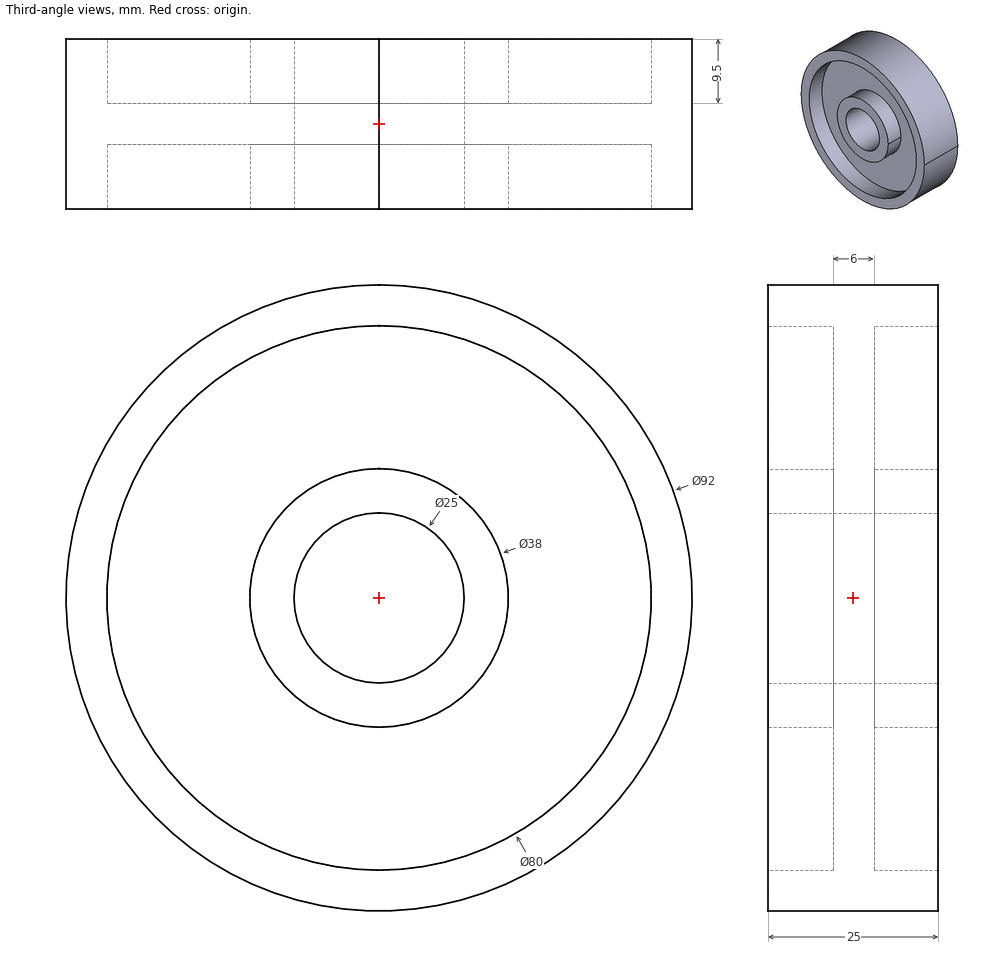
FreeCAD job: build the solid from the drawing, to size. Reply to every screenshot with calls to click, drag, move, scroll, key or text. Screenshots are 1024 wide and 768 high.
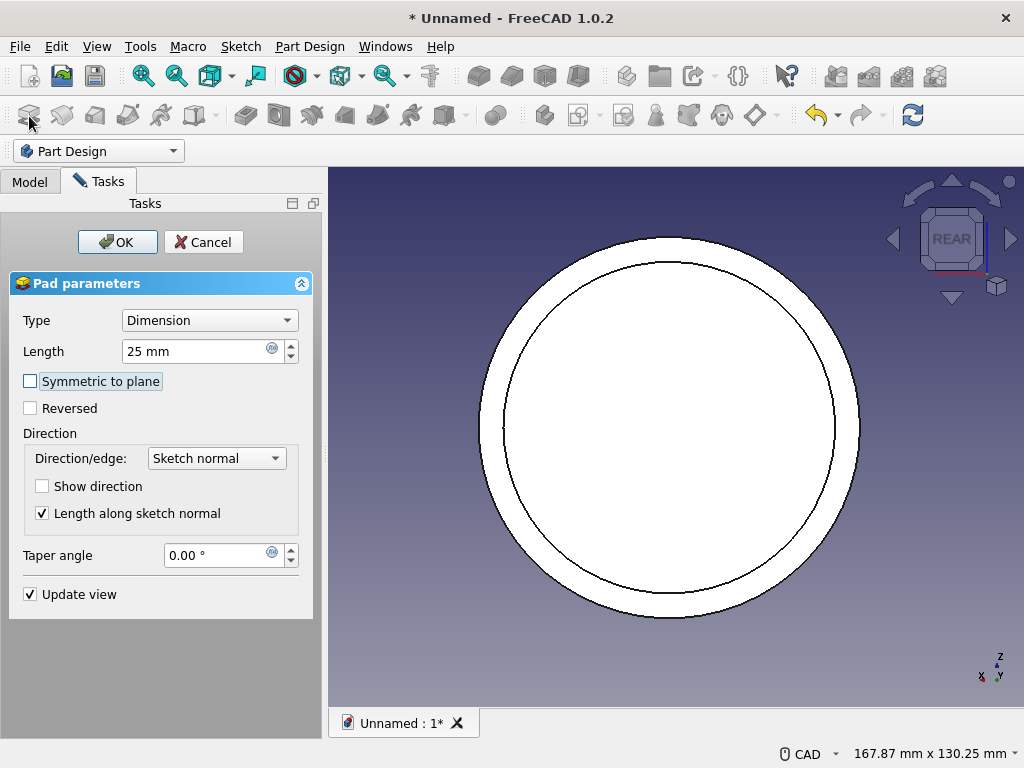
click(31, 408)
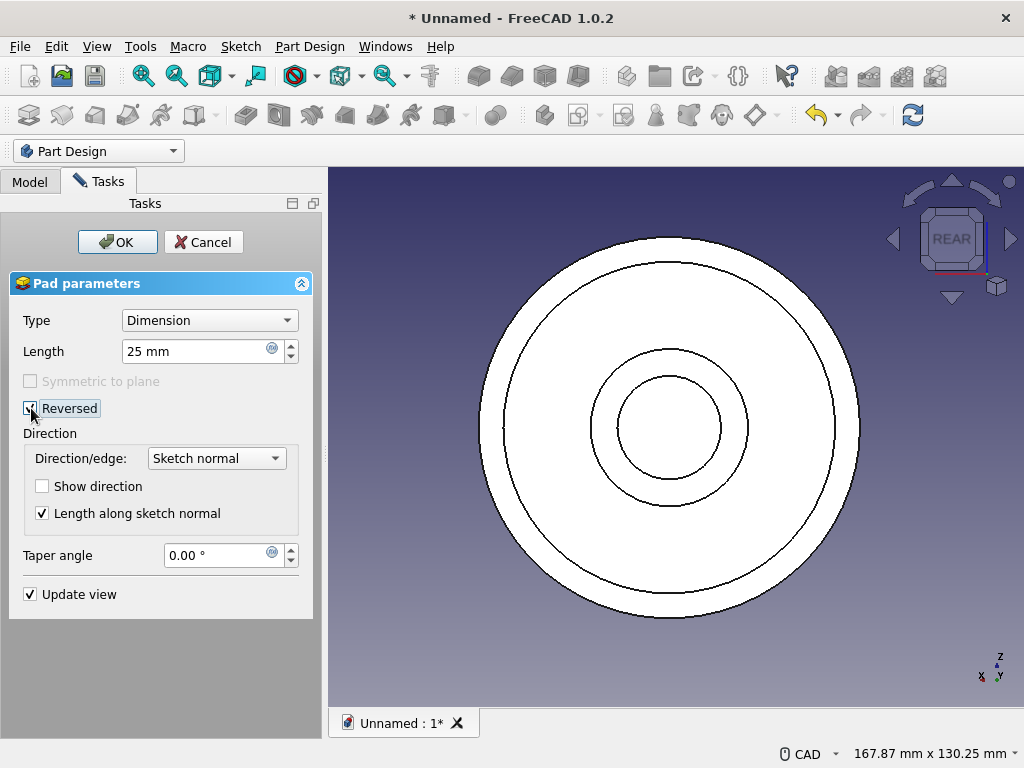
click(118, 242)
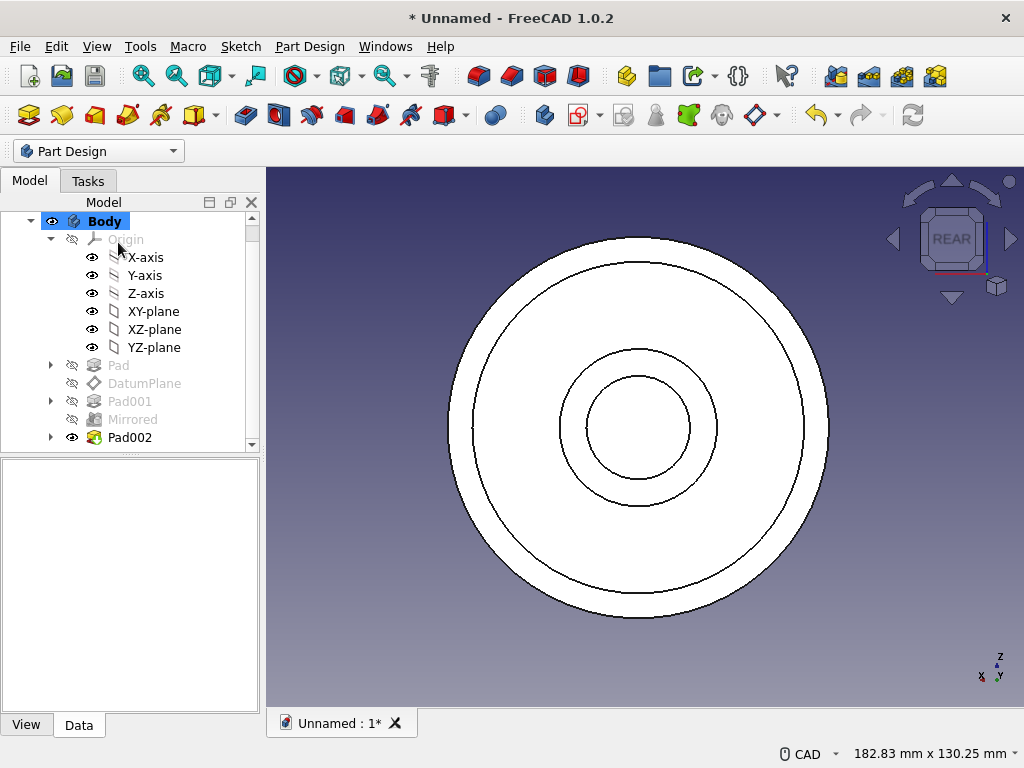
click(544, 332)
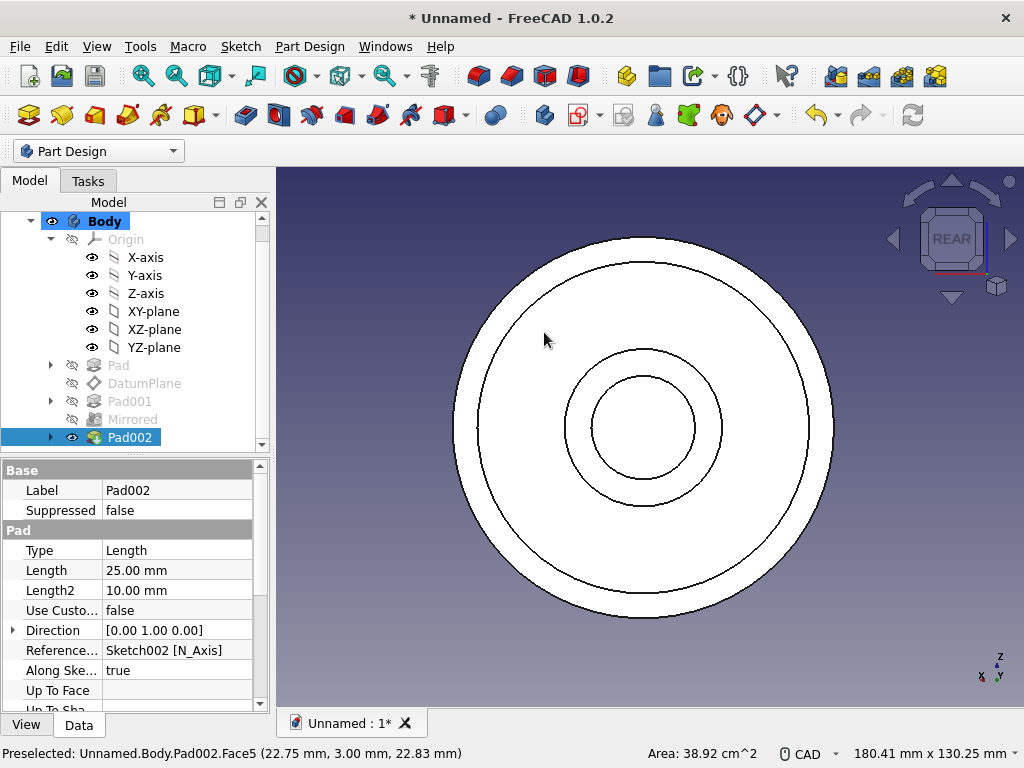
click(578, 116)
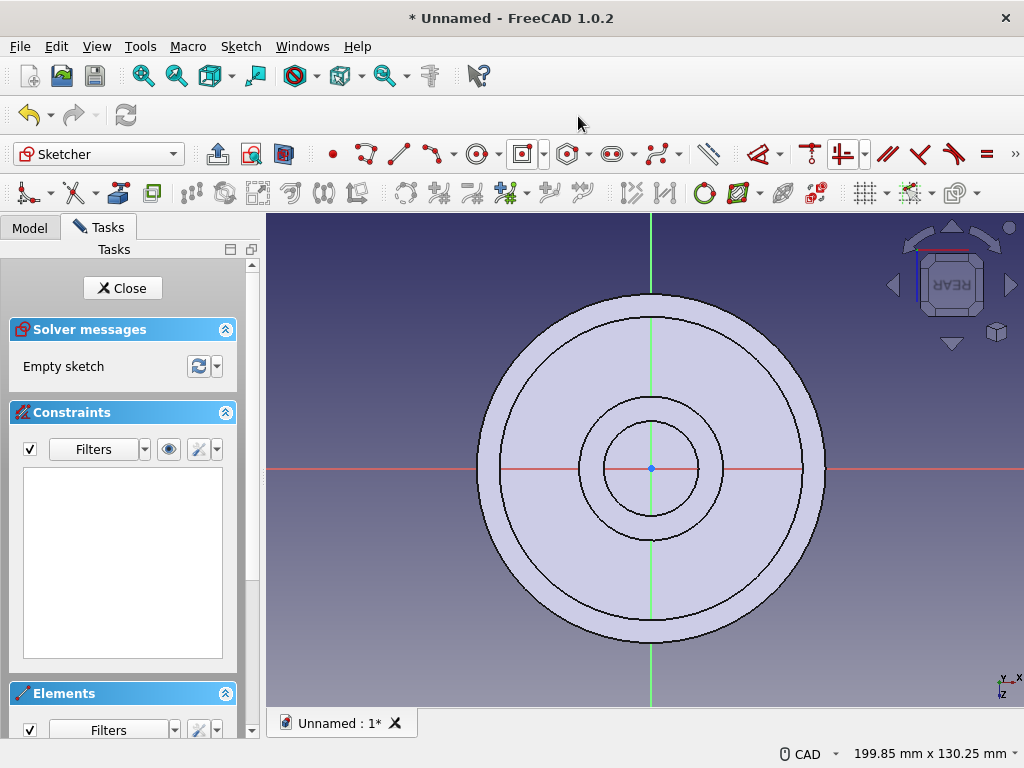
scroll(683, 472, up, 6)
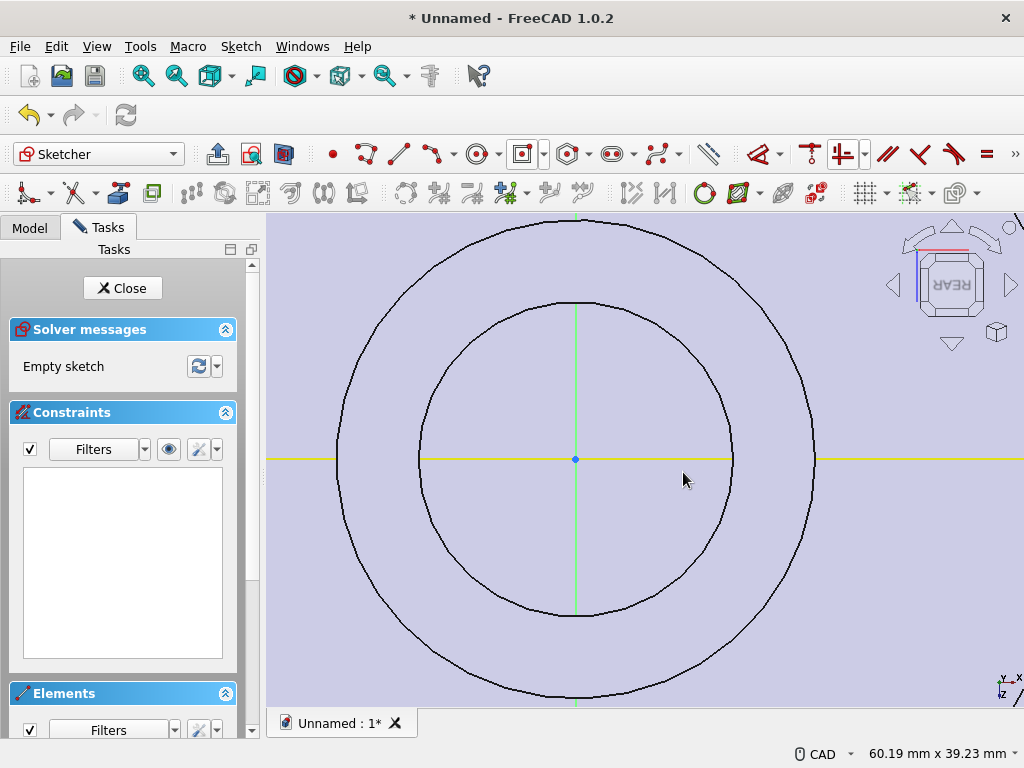
click(476, 154)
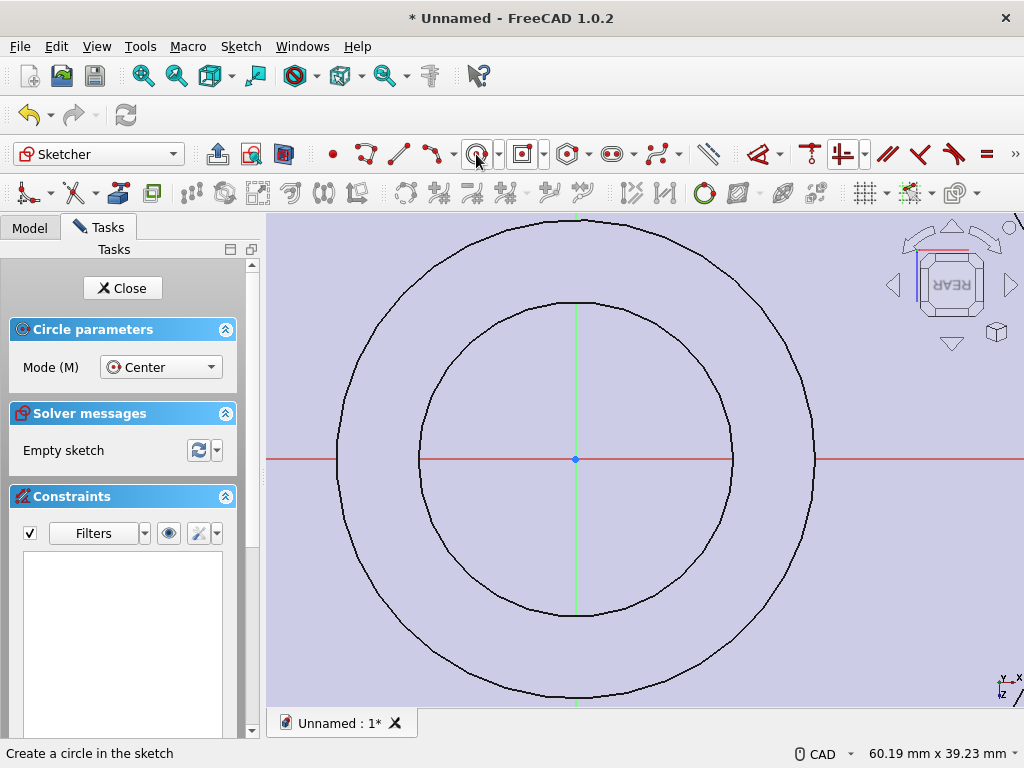
click(576, 459)
move(687, 348)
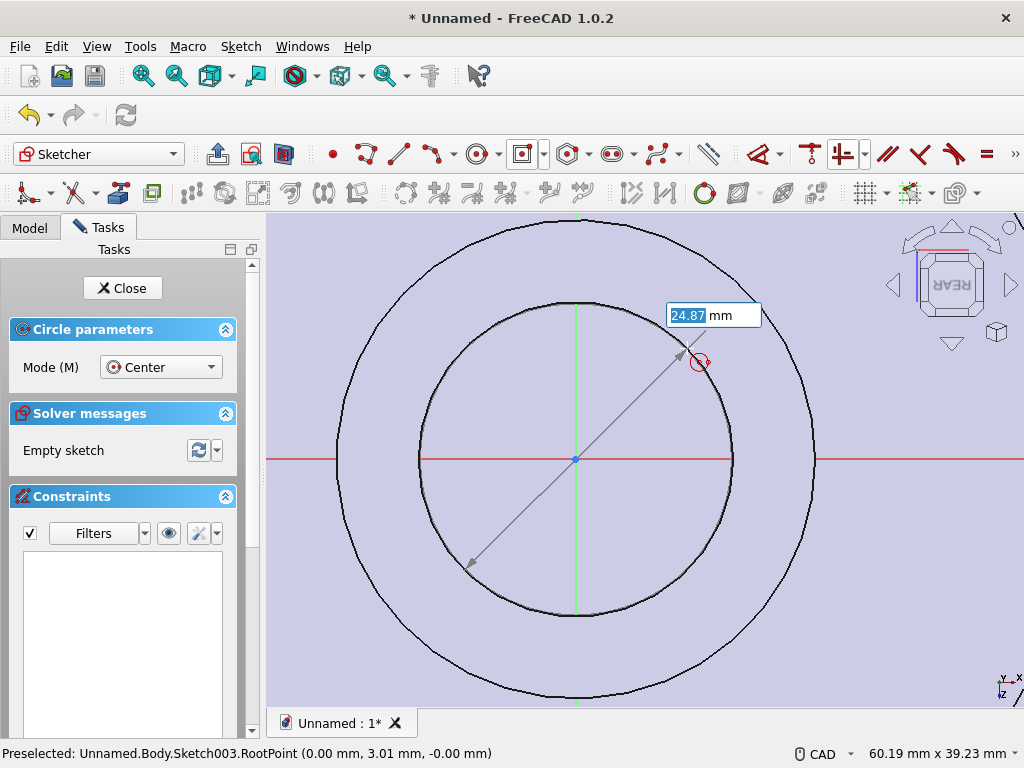
text(25)
key(Return)
key(Escape)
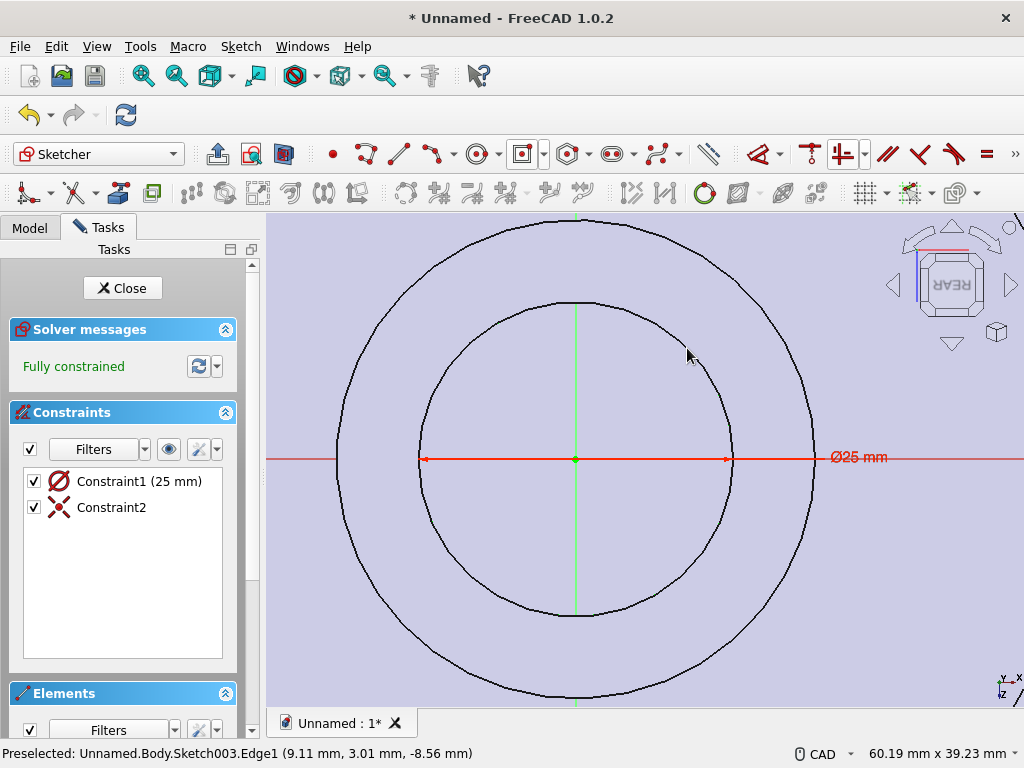
click(123, 288)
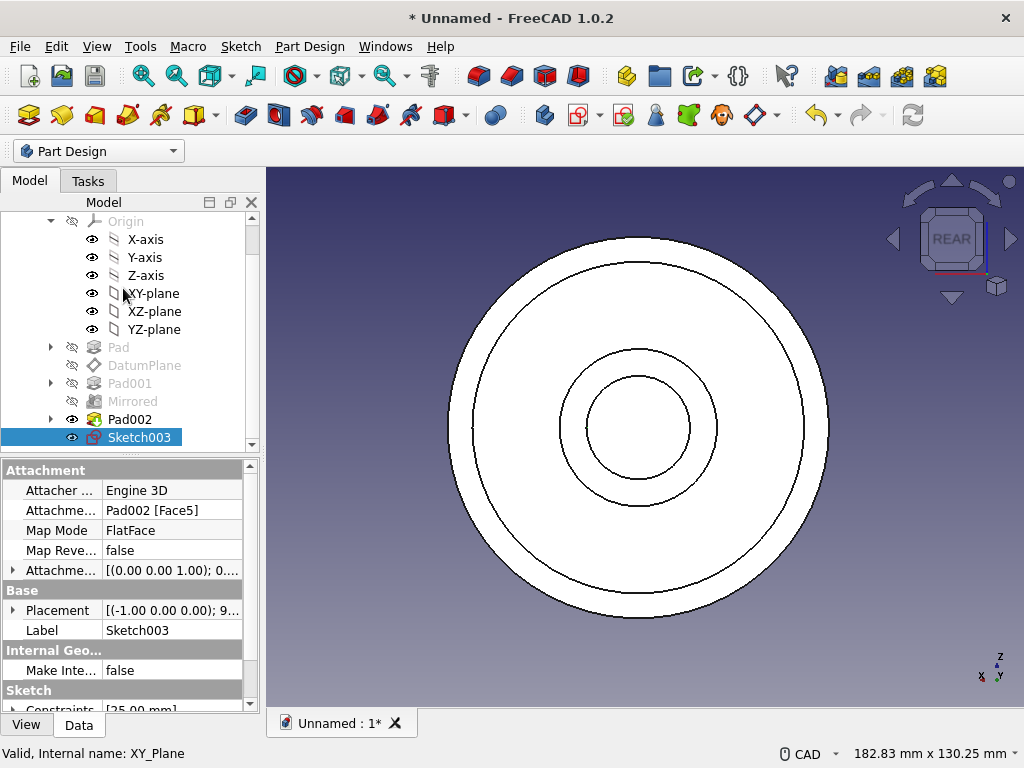
click(246, 116)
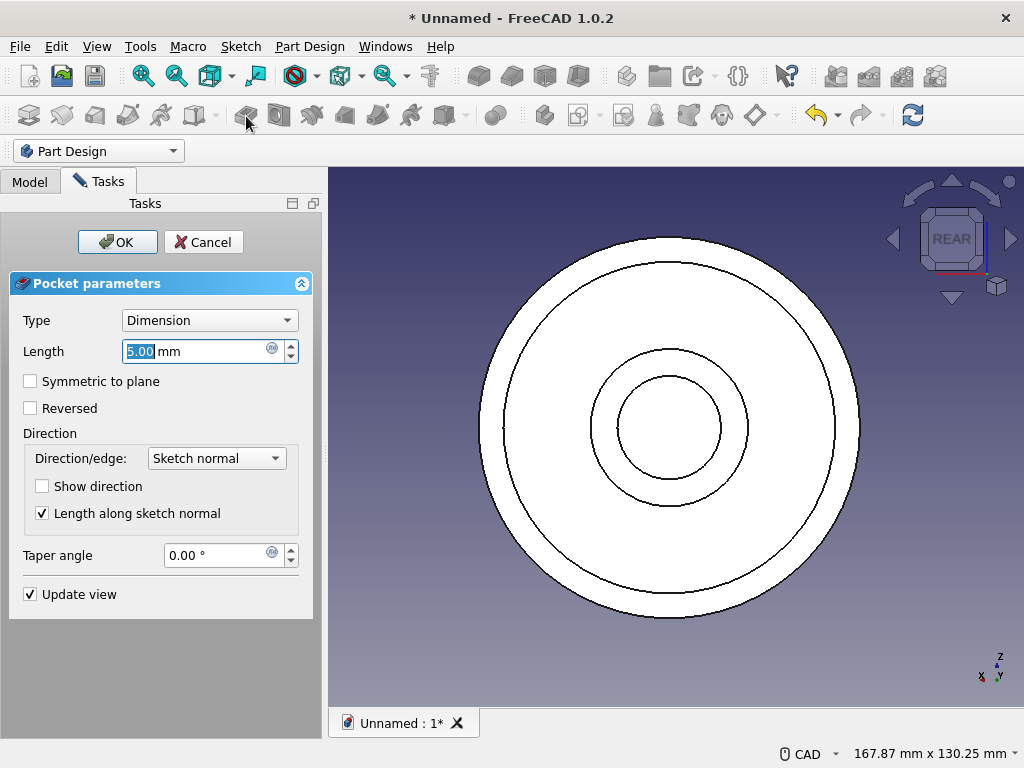
text(25)
key(Tab)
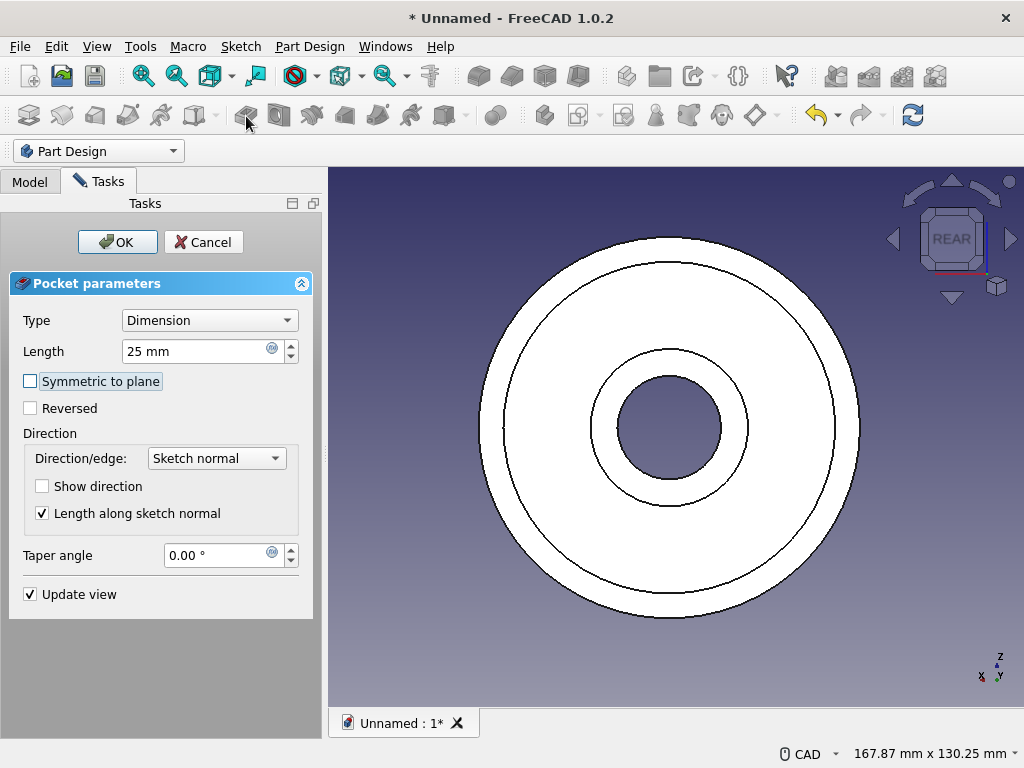
click(118, 242)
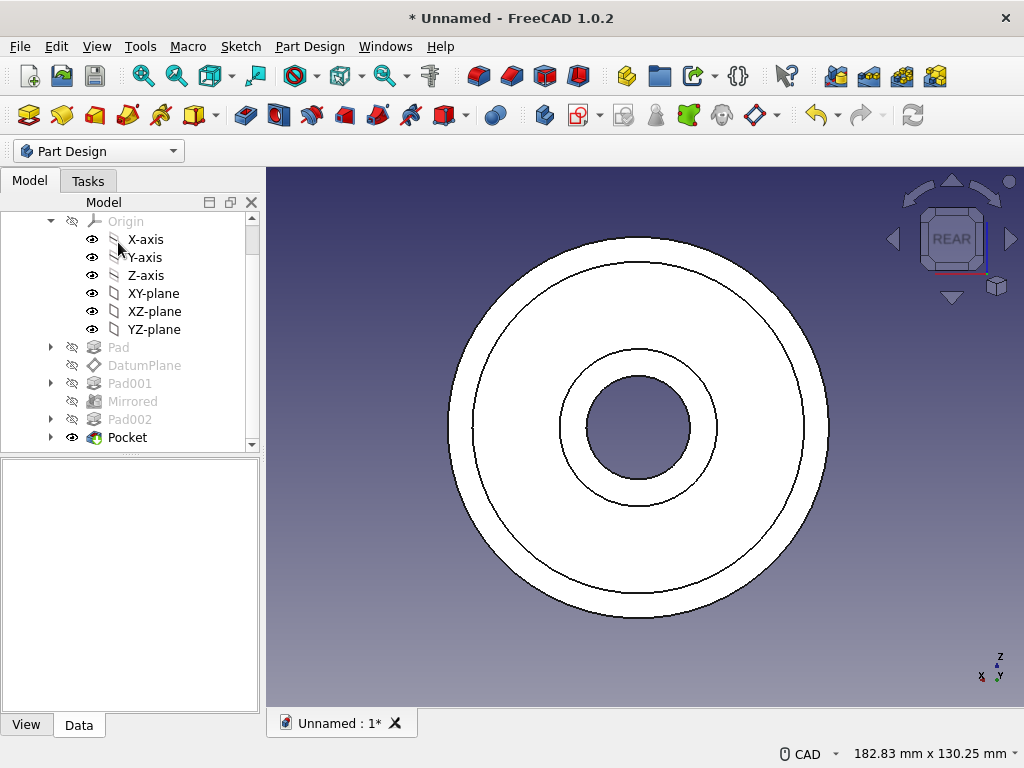
key(0)